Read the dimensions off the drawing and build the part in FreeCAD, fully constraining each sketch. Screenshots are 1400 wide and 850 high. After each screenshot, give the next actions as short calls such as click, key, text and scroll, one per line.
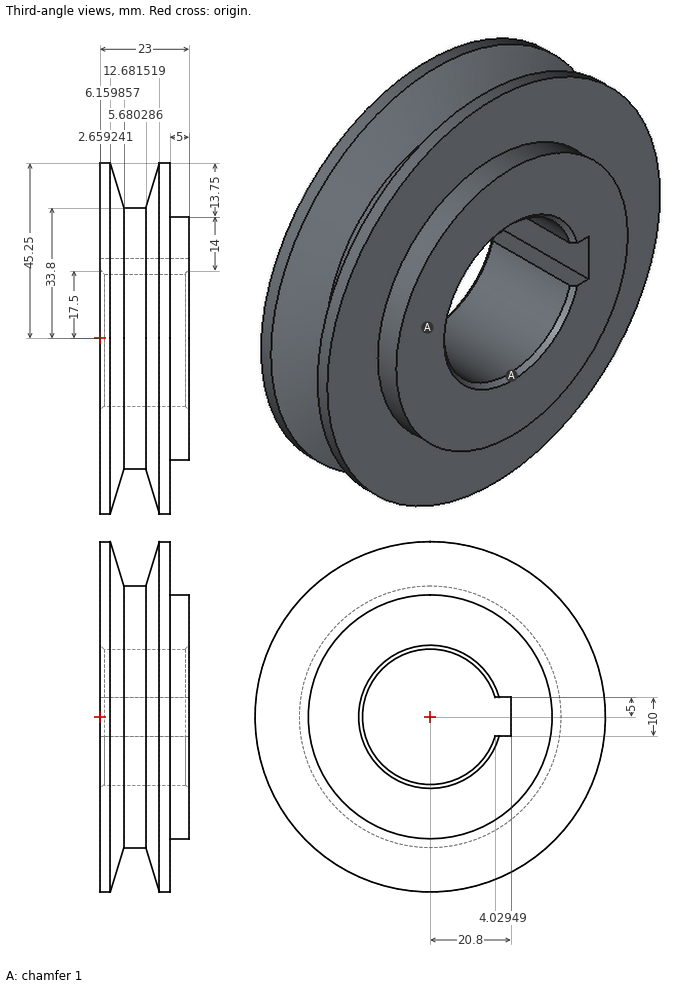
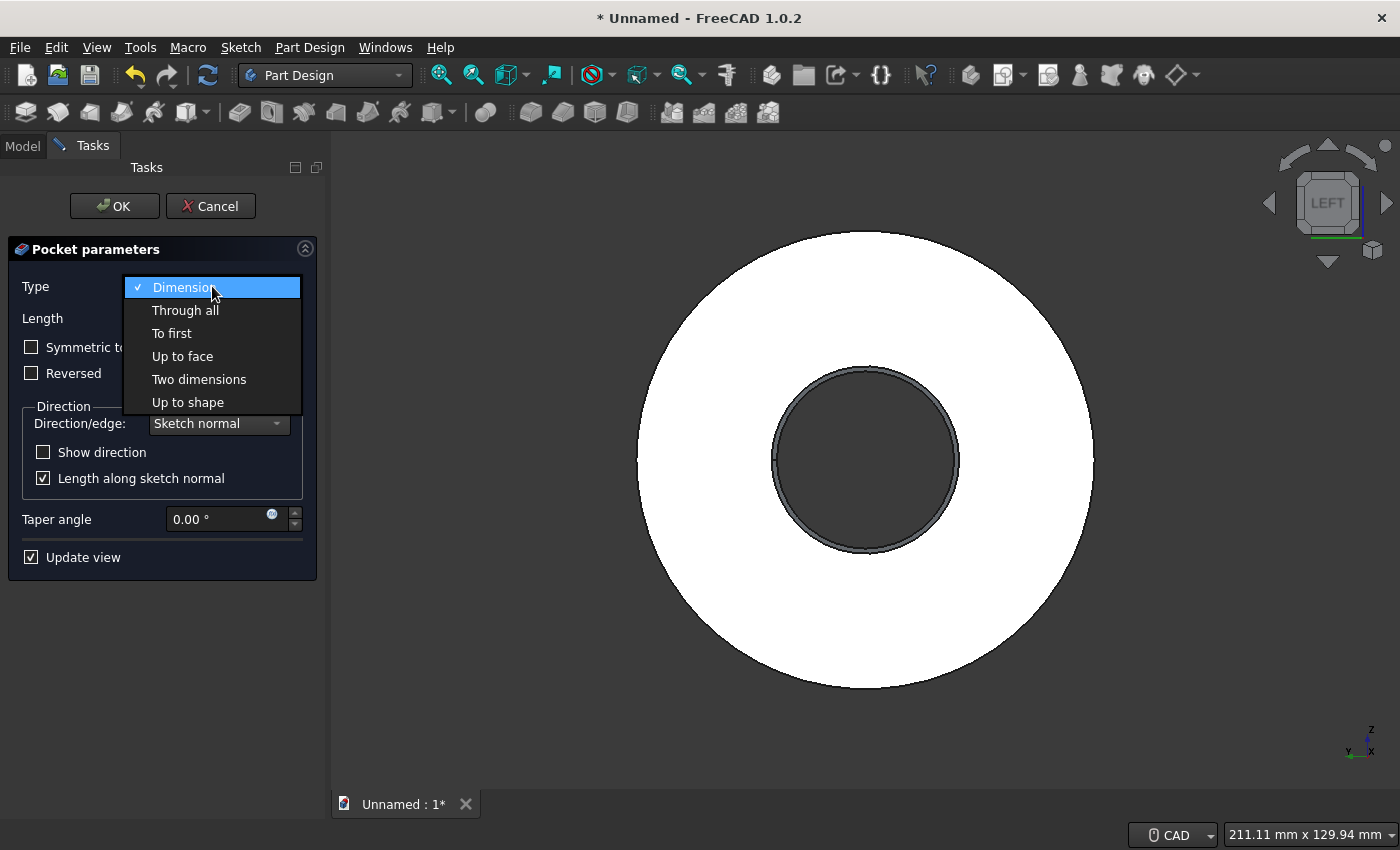
click(212, 310)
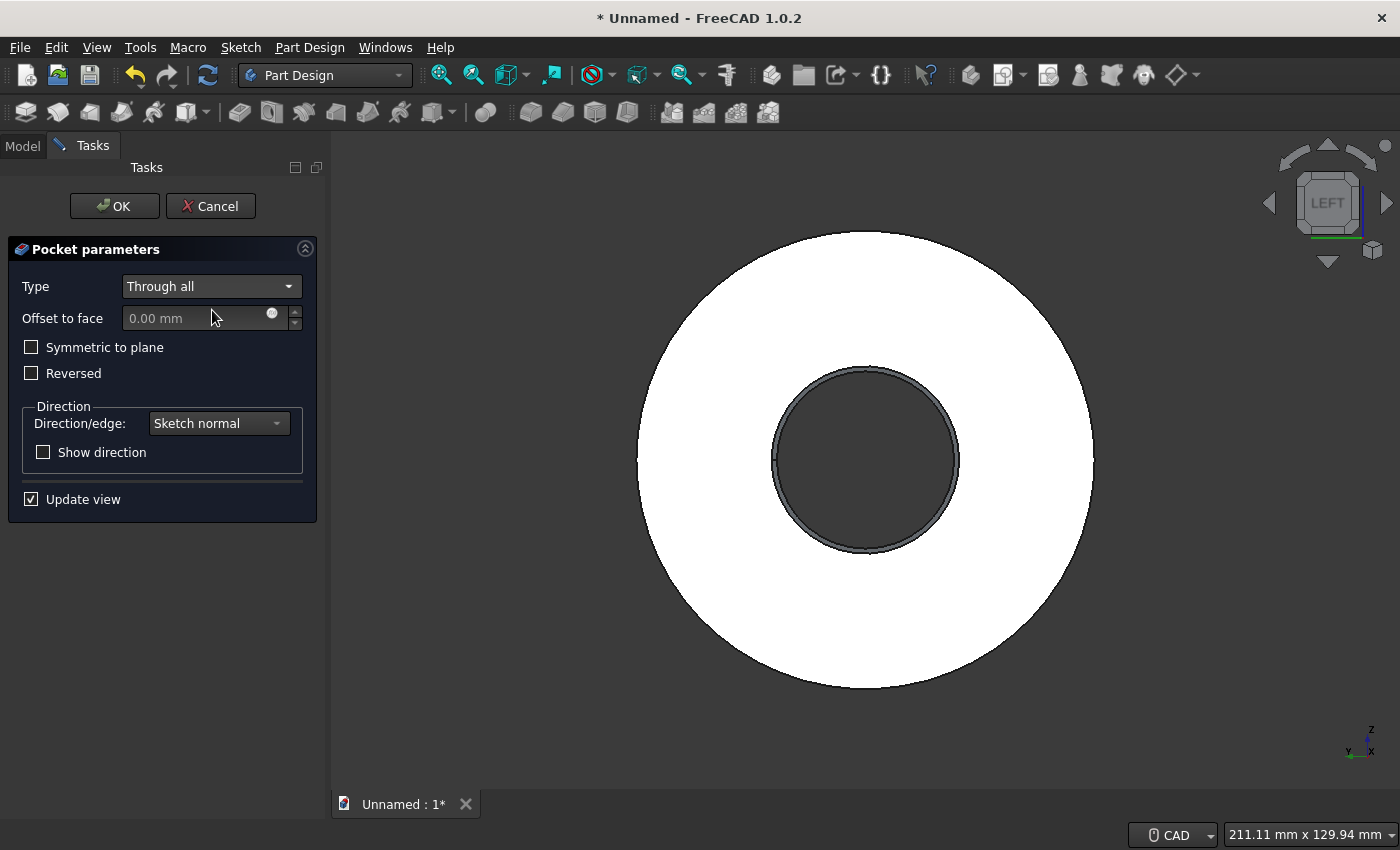
click(30, 373)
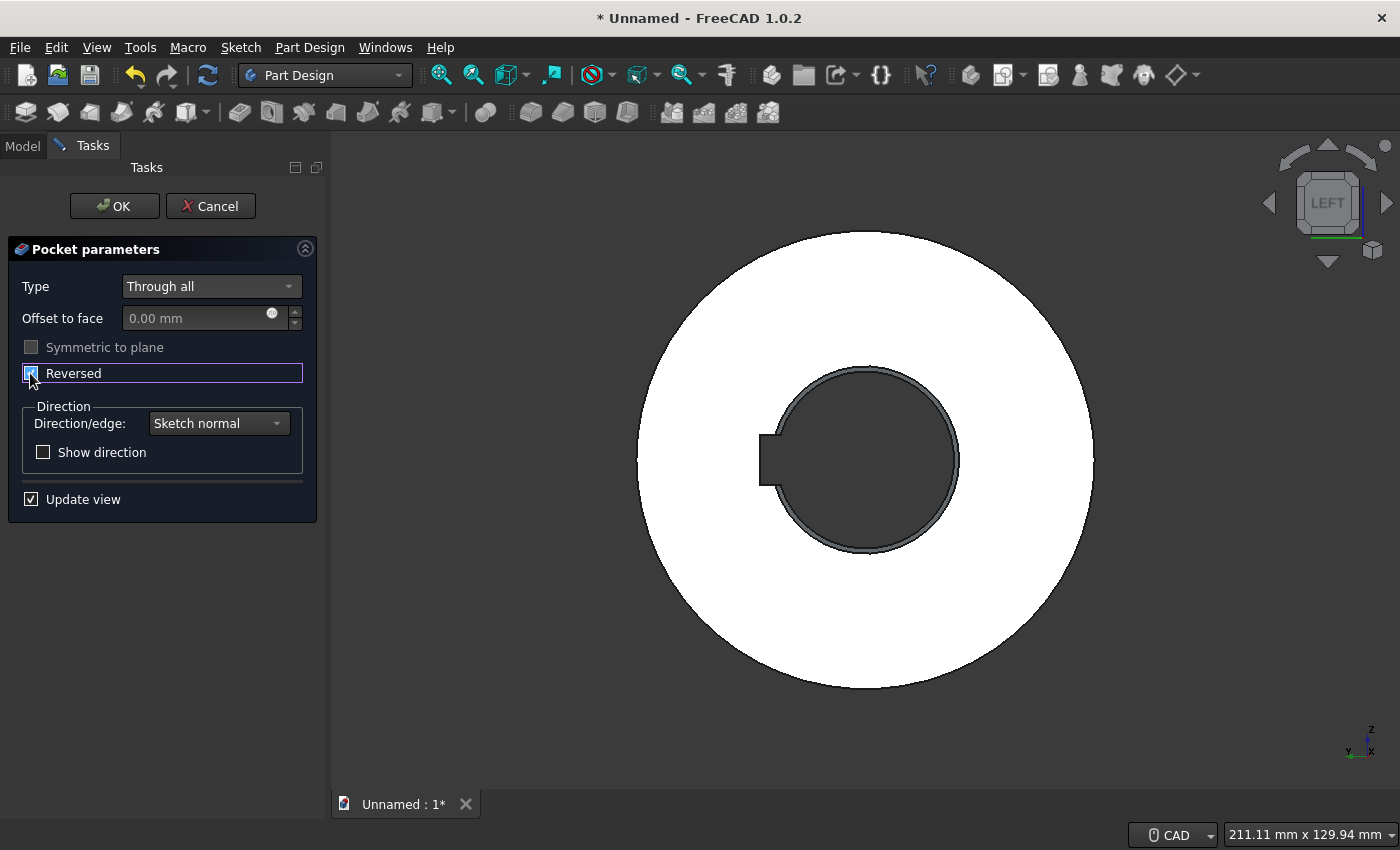
click(115, 206)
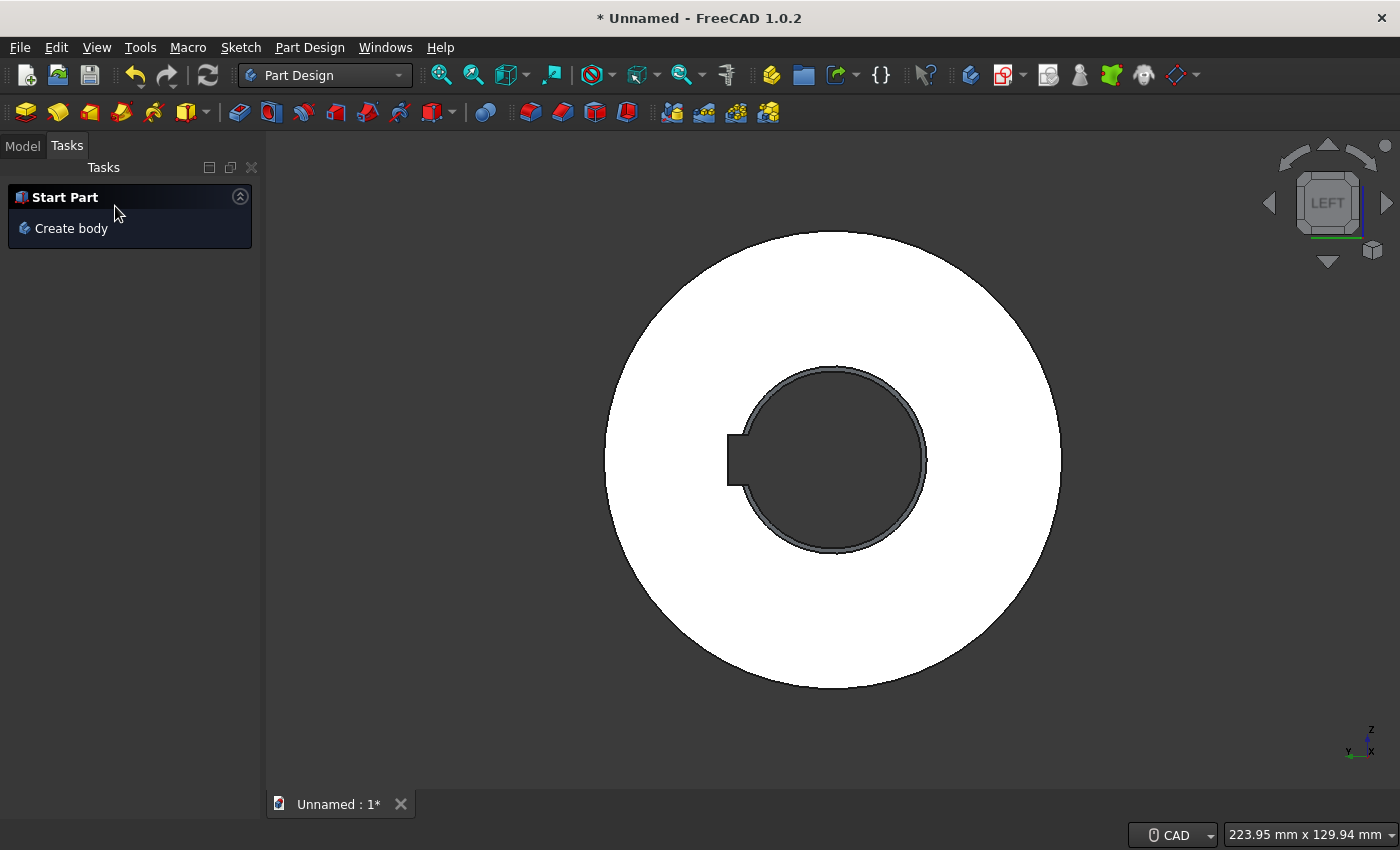
key(0)